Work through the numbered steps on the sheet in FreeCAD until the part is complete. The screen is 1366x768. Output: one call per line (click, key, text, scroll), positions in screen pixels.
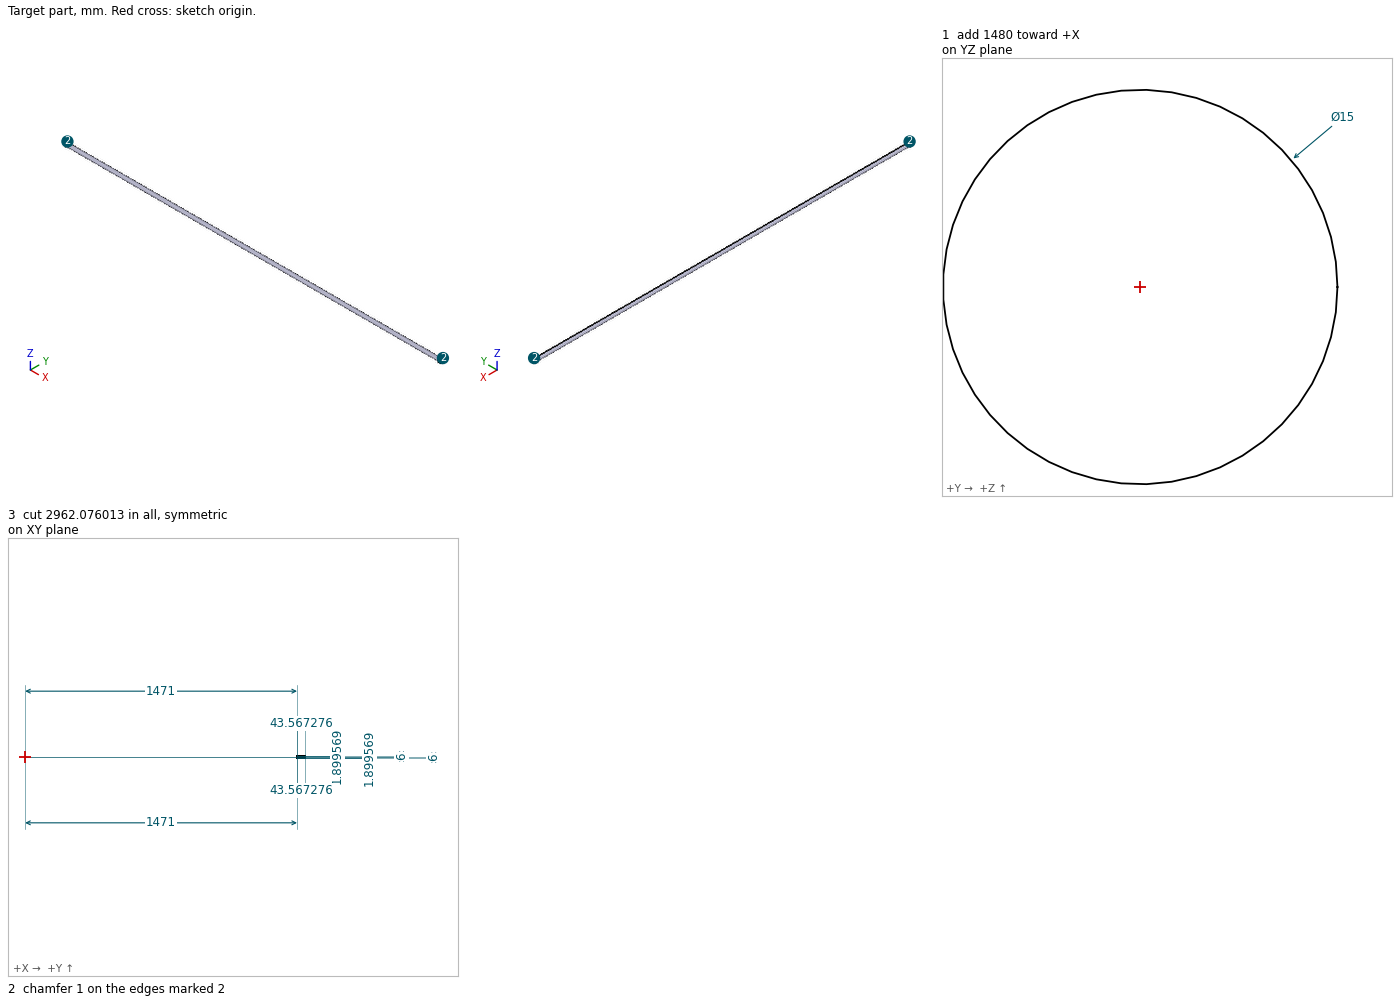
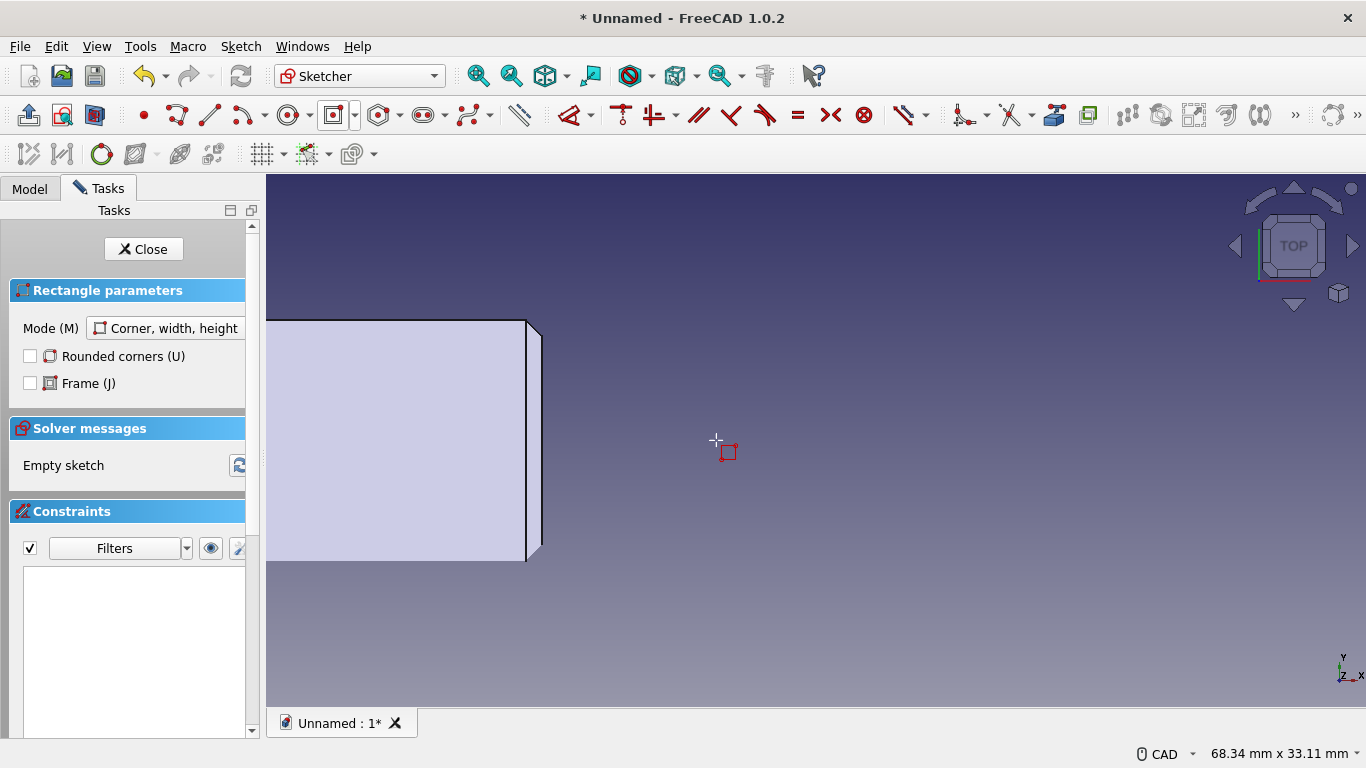
click(397, 313)
click(1098, 344)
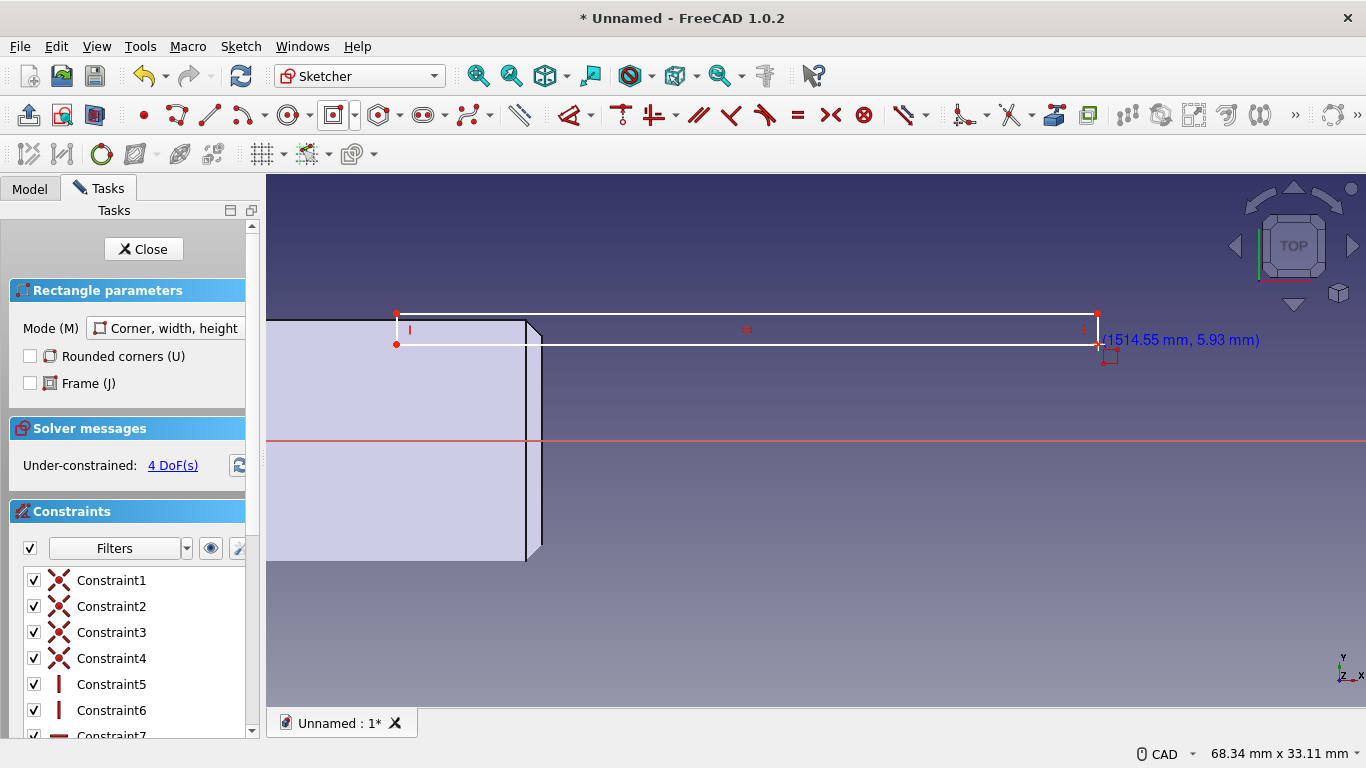
click(397, 537)
click(1098, 568)
key(Escape)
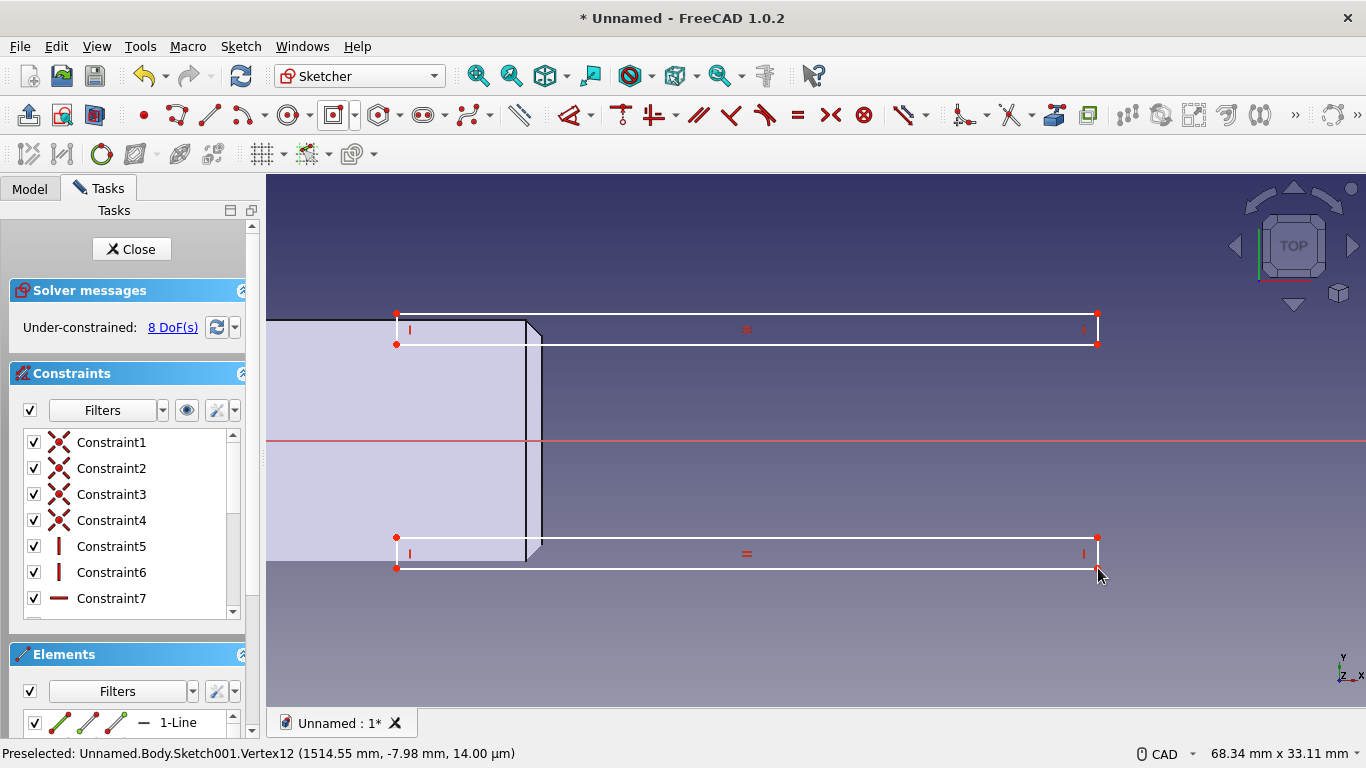
click(568, 116)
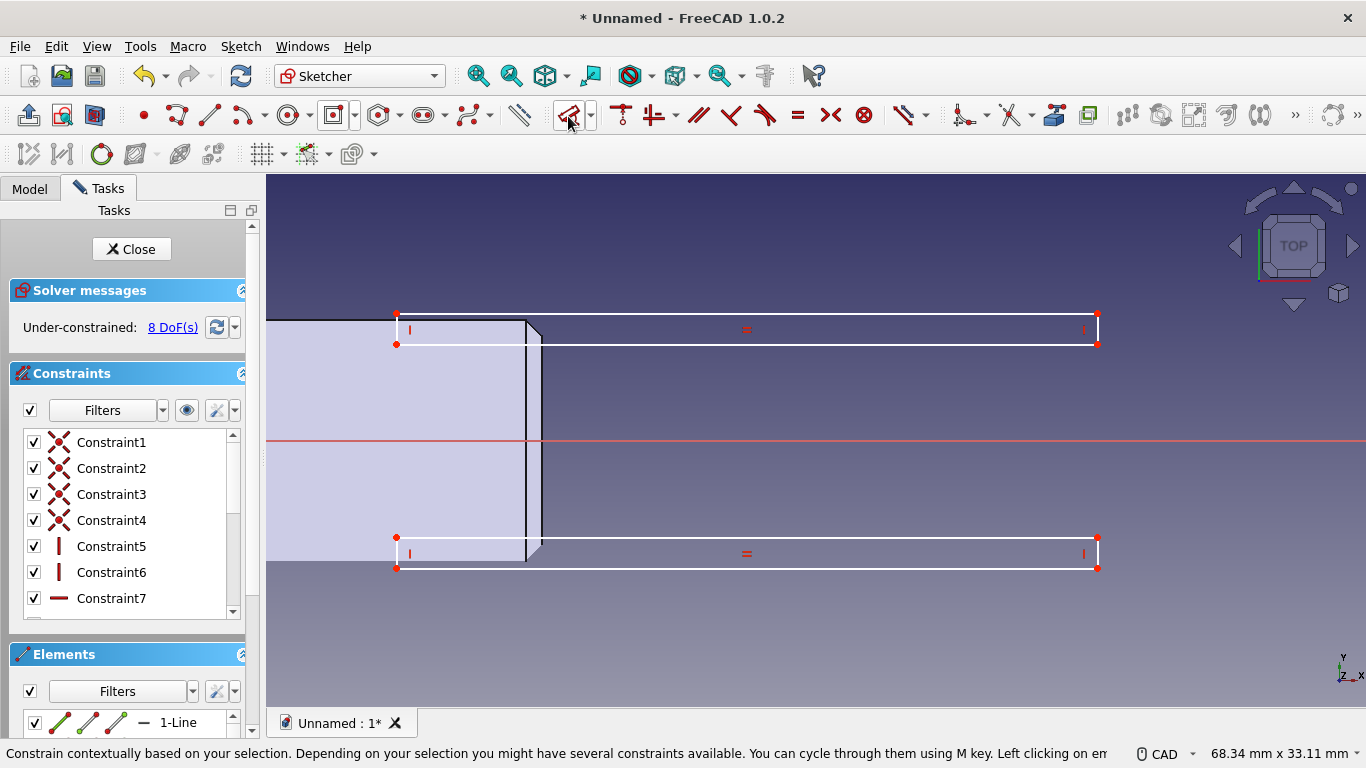
click(397, 345)
click(431, 393)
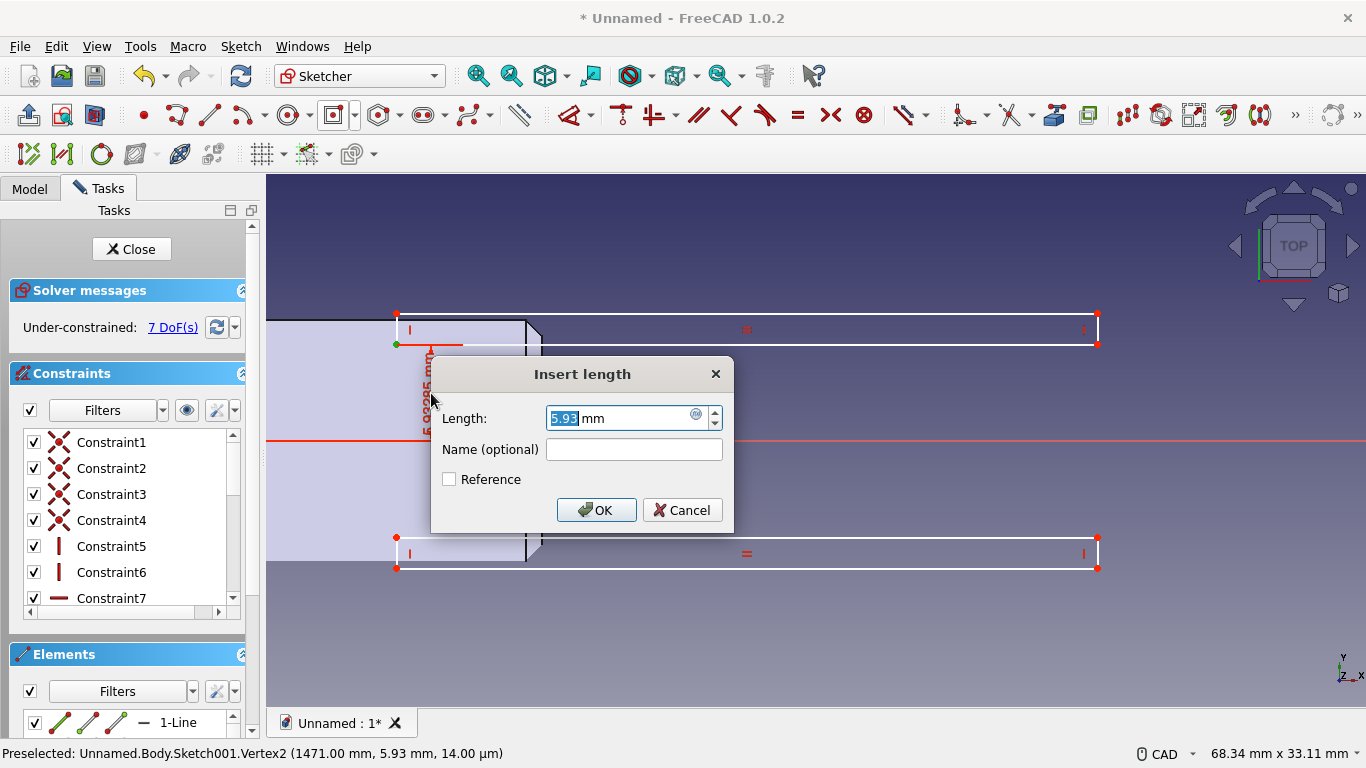
text(6)
key(Return)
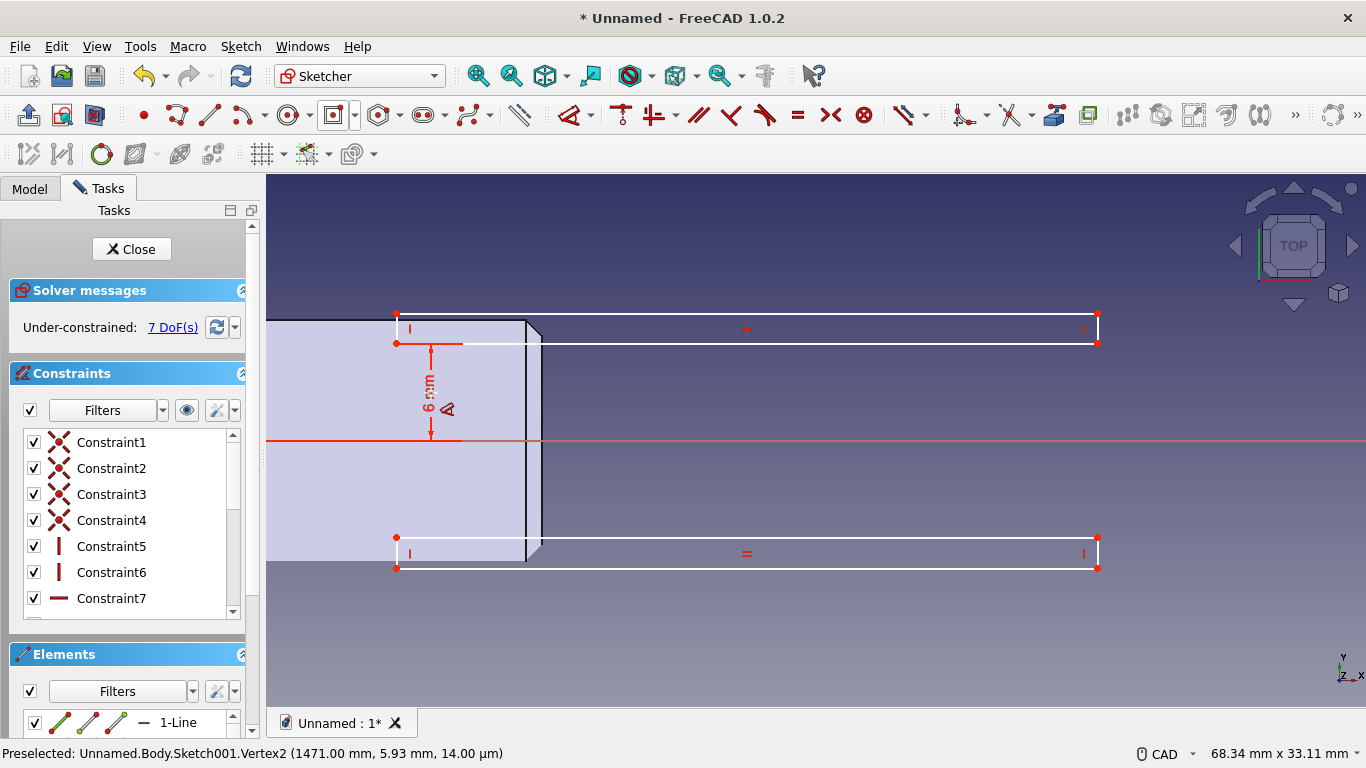
click(397, 538)
click(431, 489)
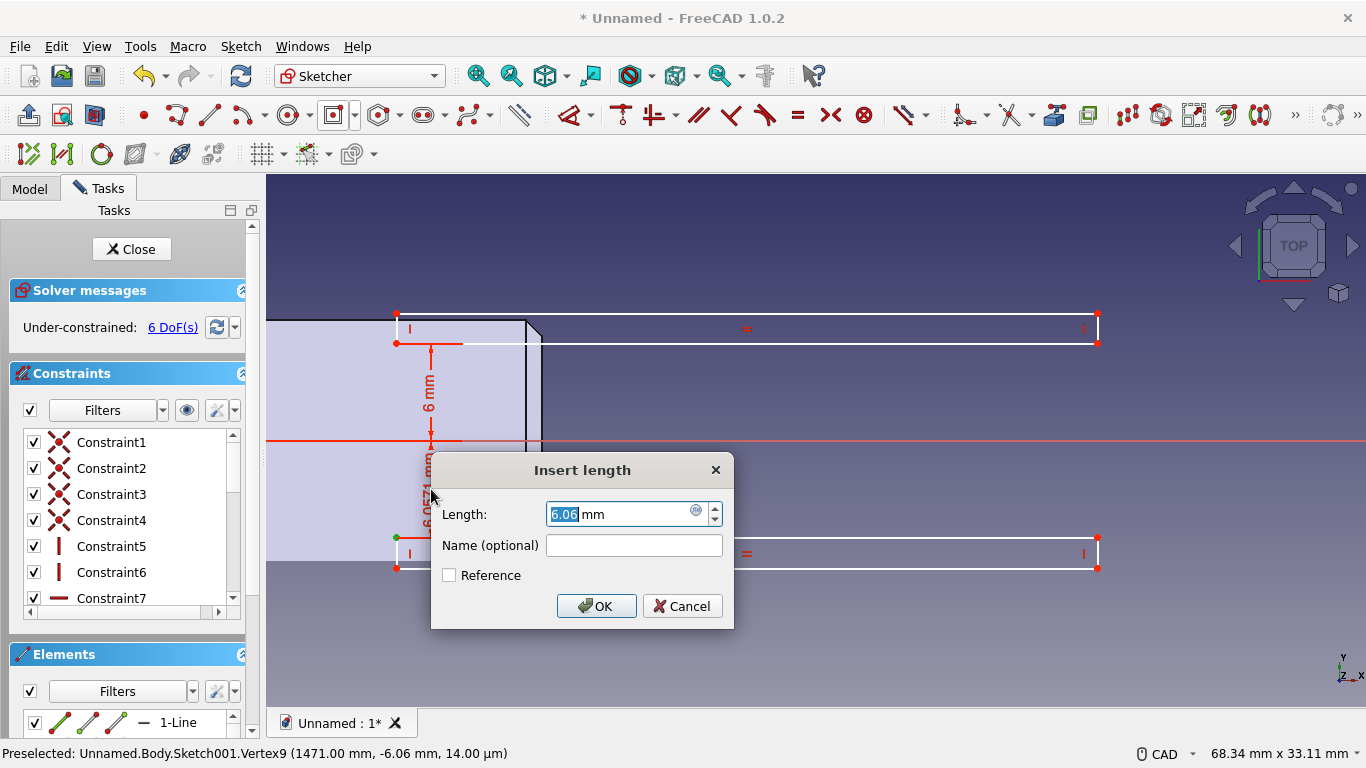
text(6)
key(Return)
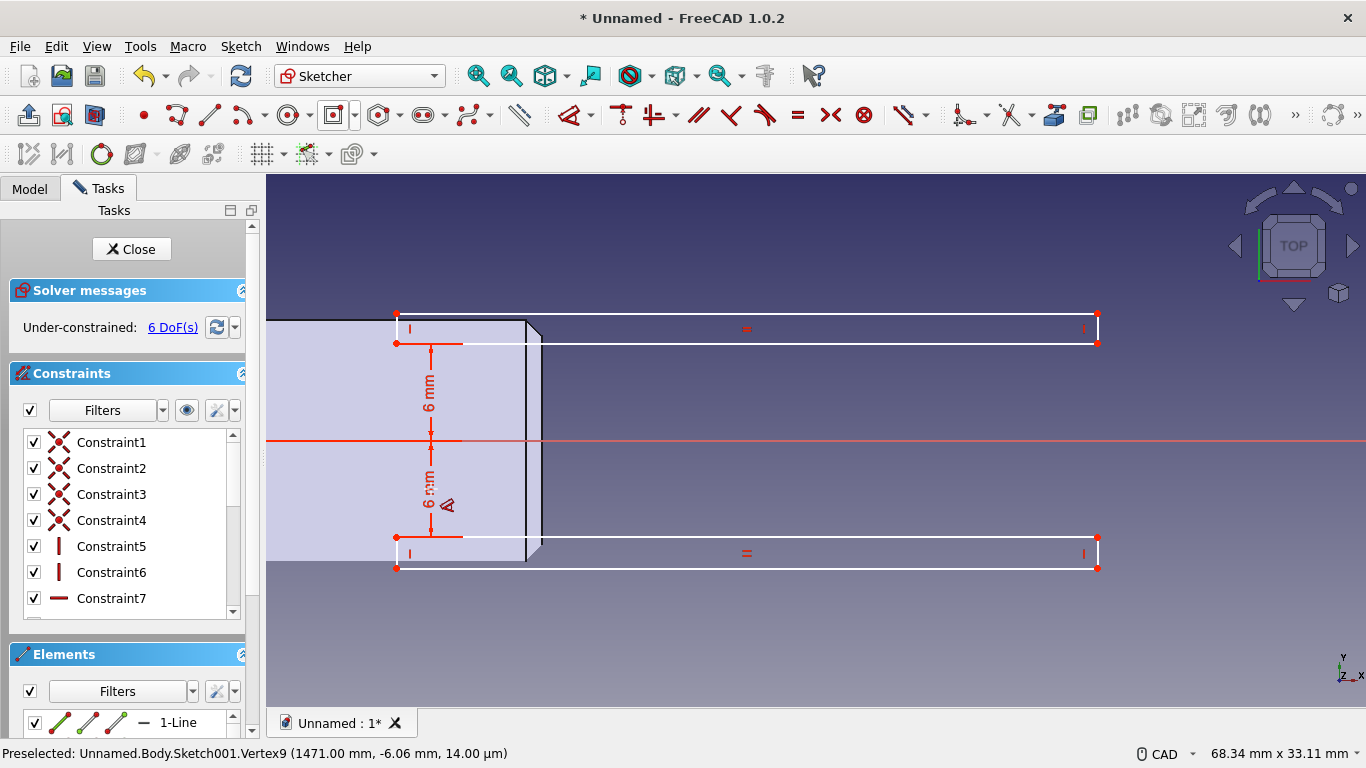
click(397, 314)
click(345, 280)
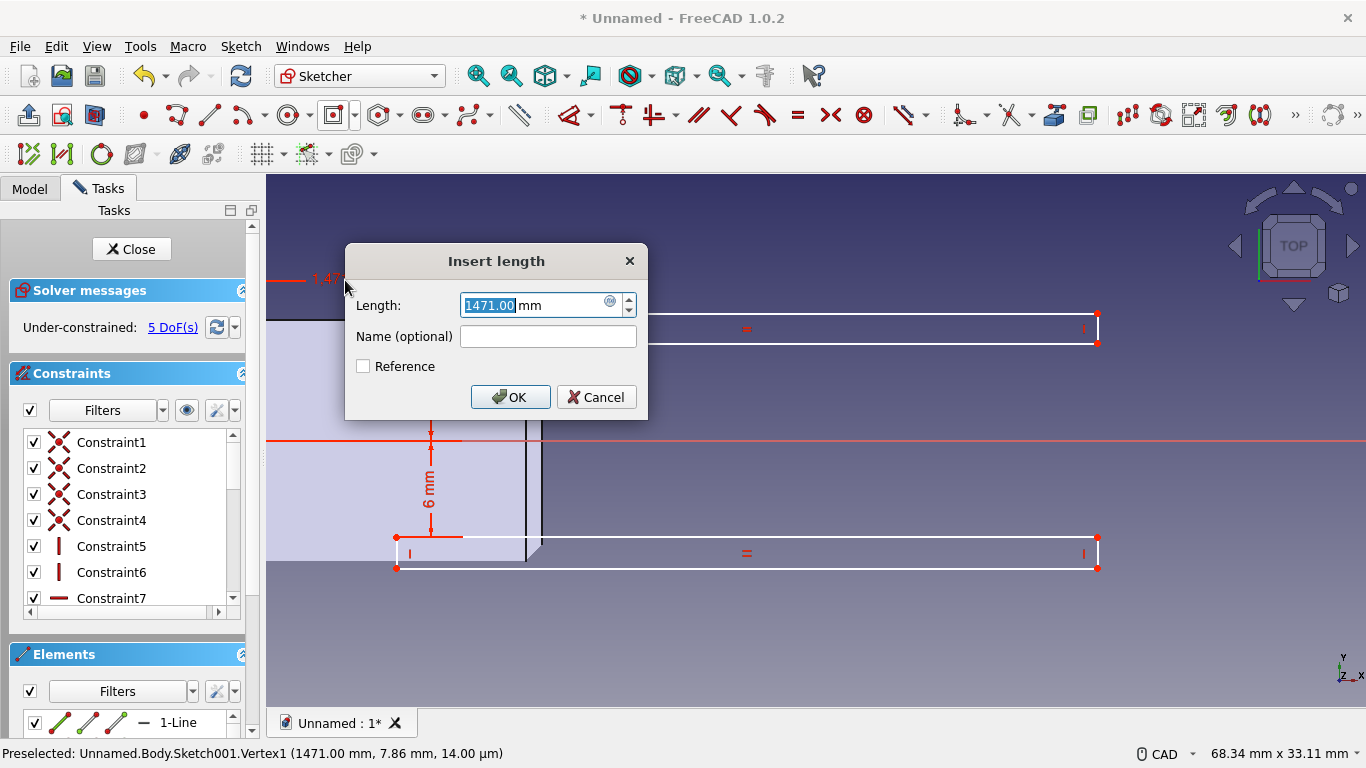
text(1471)
key(Return)